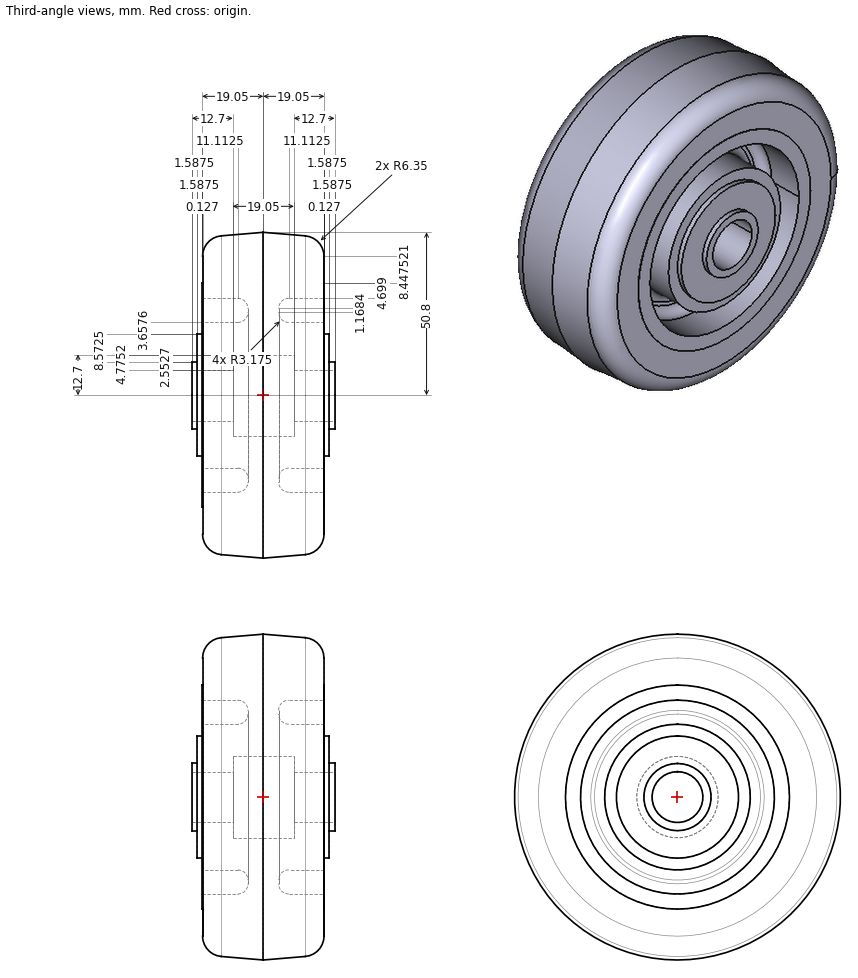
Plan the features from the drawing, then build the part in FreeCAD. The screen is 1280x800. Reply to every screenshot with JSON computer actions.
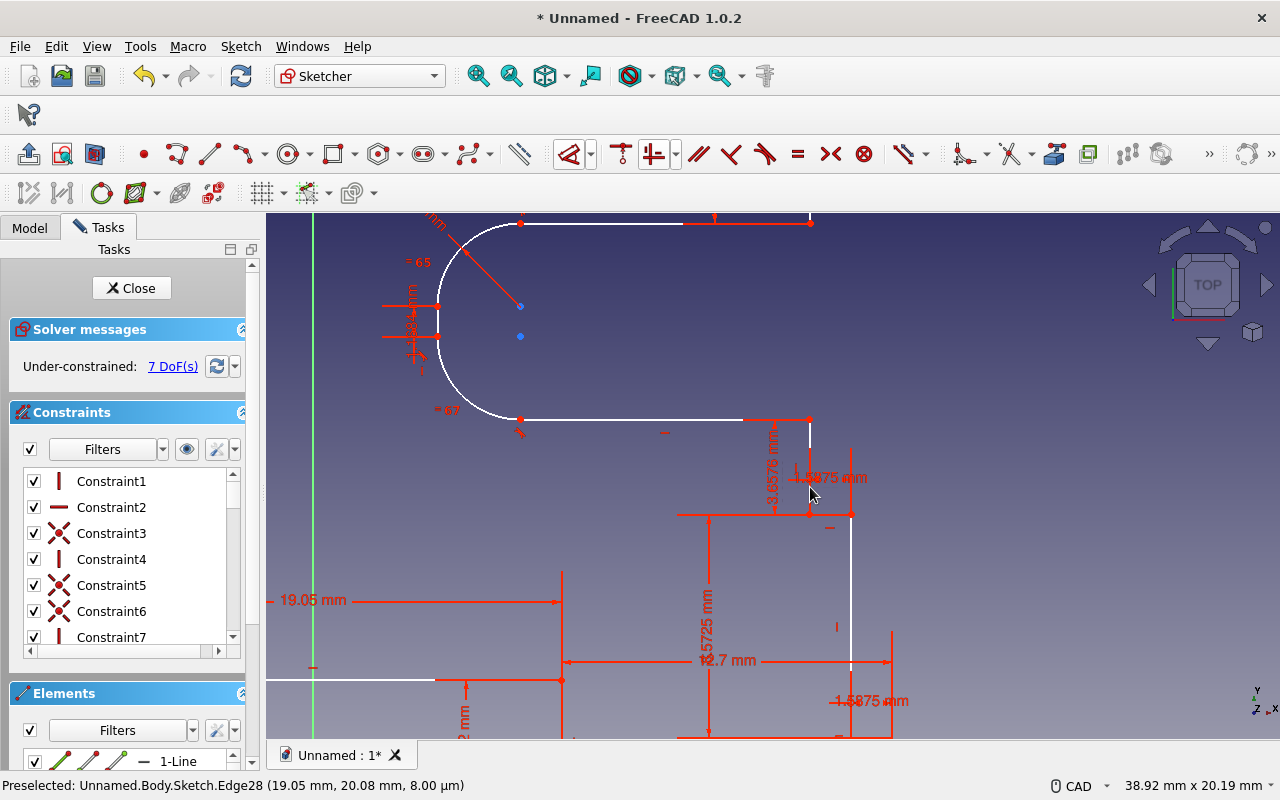
{"action": "scroll", "coordinate": [832, 517], "scroll_direction": "down", "scroll_amount": 7}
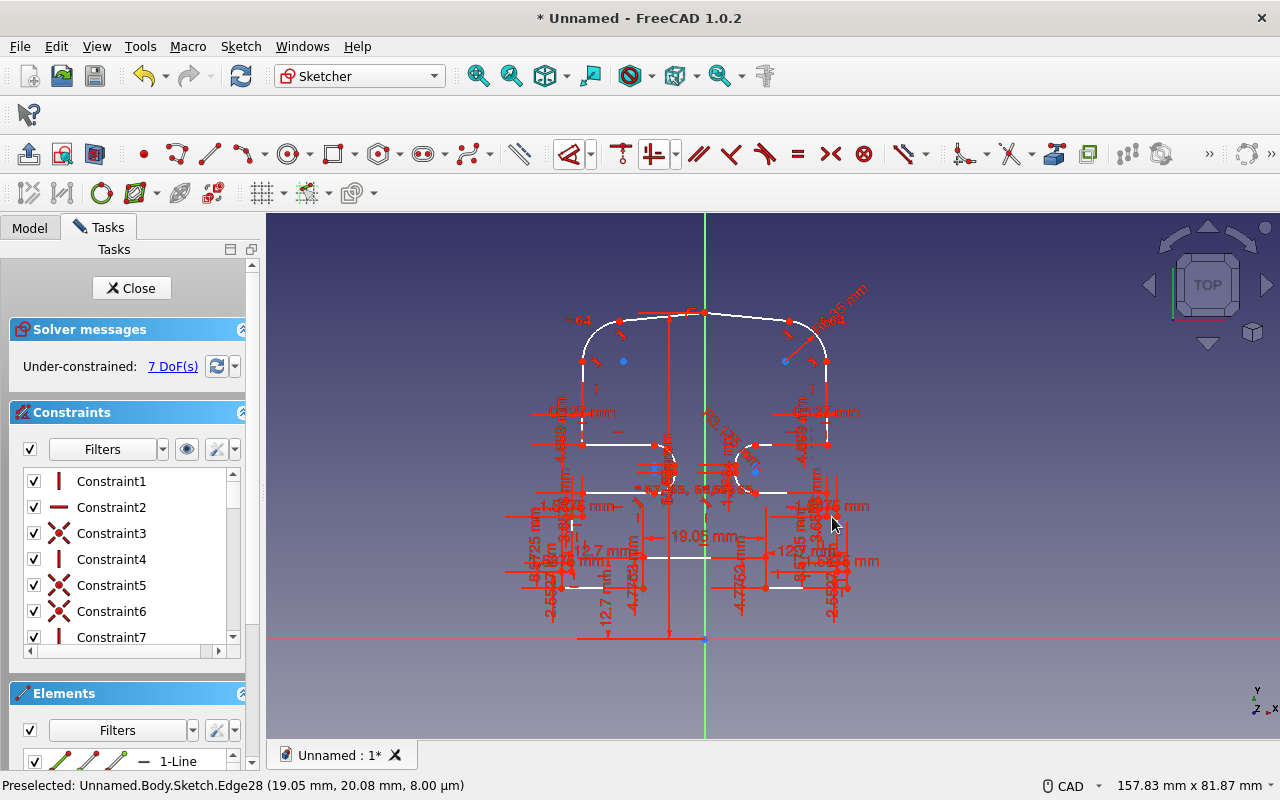
{"action": "left_click", "coordinate": [827, 445]}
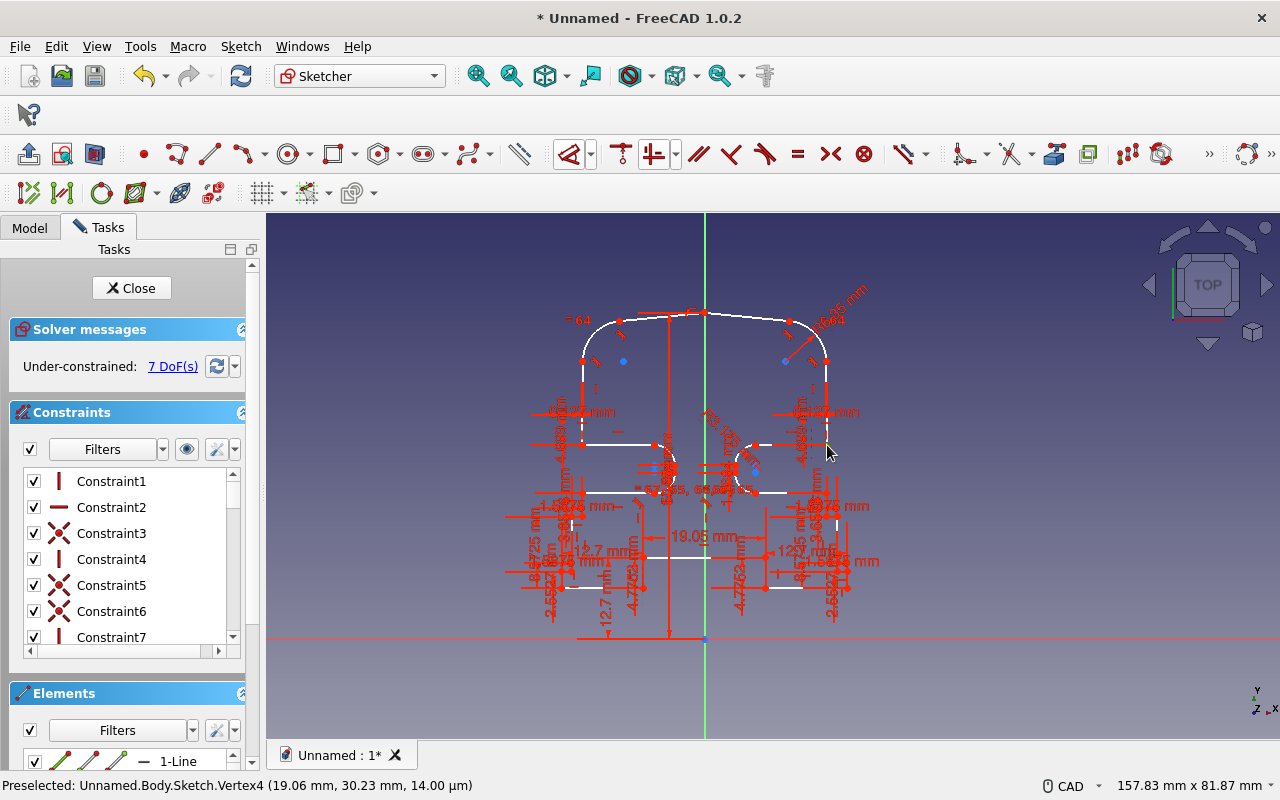
{"action": "left_click", "coordinate": [590, 154]}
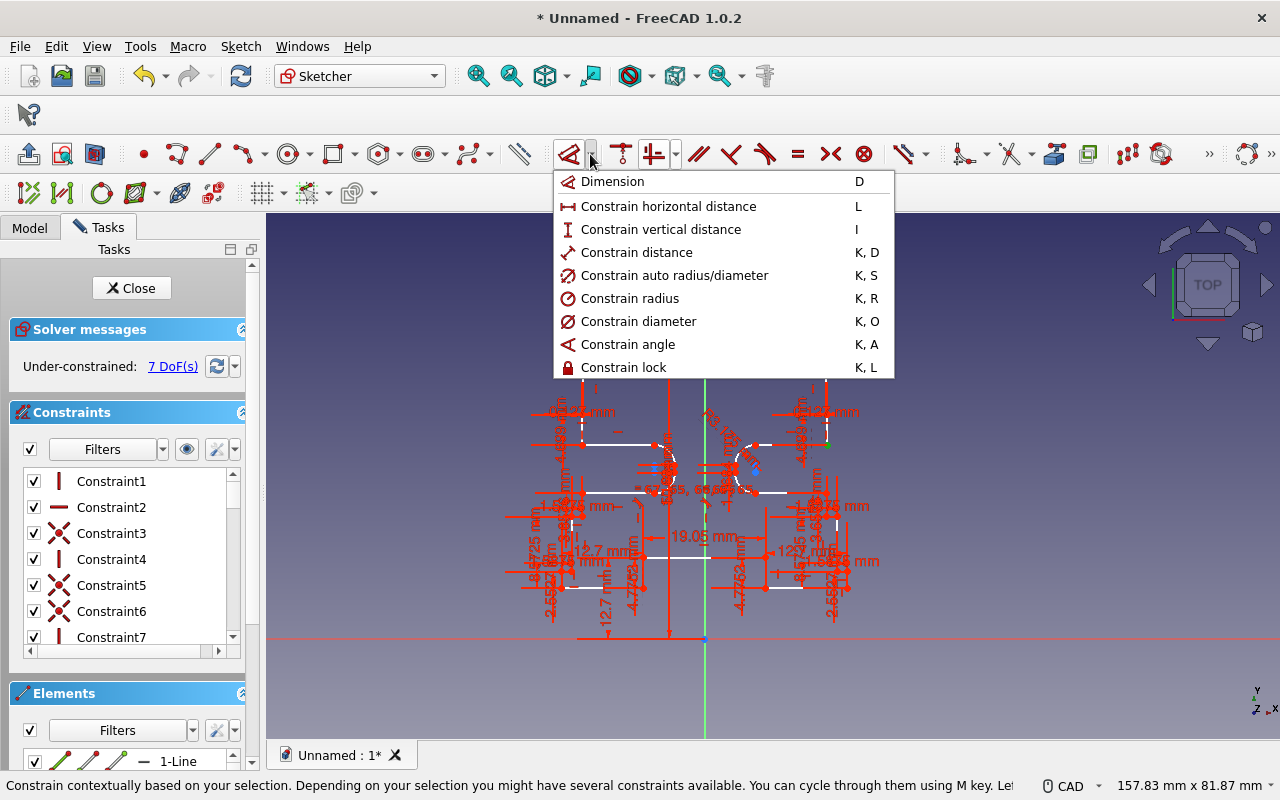
{"action": "left_click", "coordinate": [724, 206]}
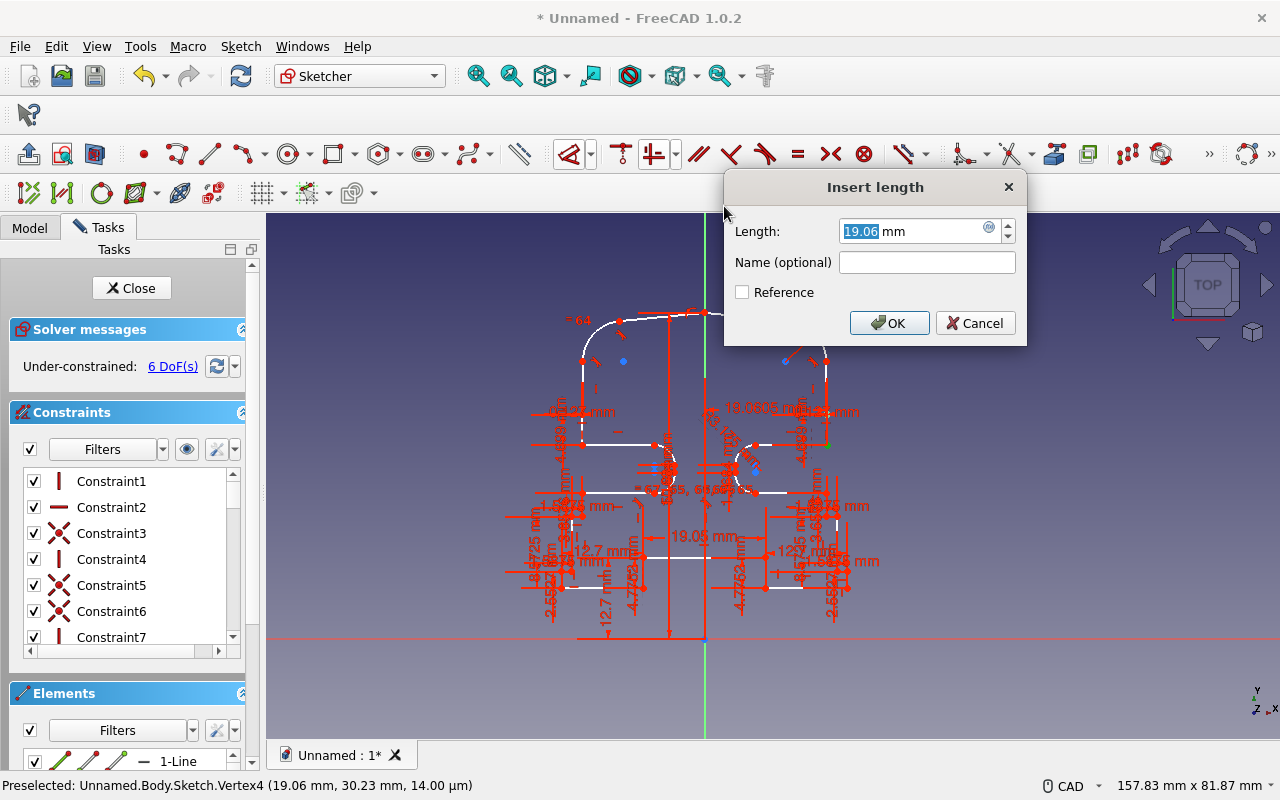
{"action": "type", "text": "19.05"}
{"action": "key", "text": "Return"}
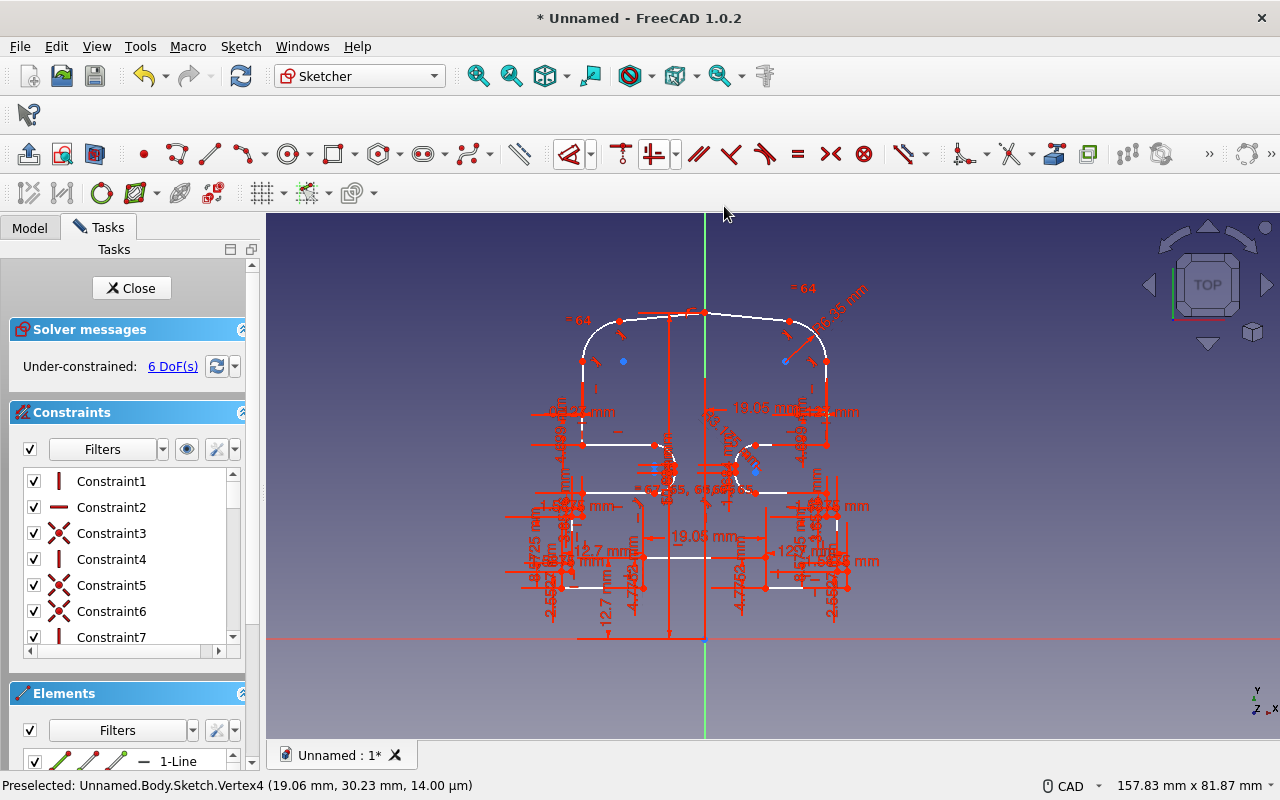
{"action": "scroll", "coordinate": [582, 415], "scroll_direction": "up", "scroll_amount": 14}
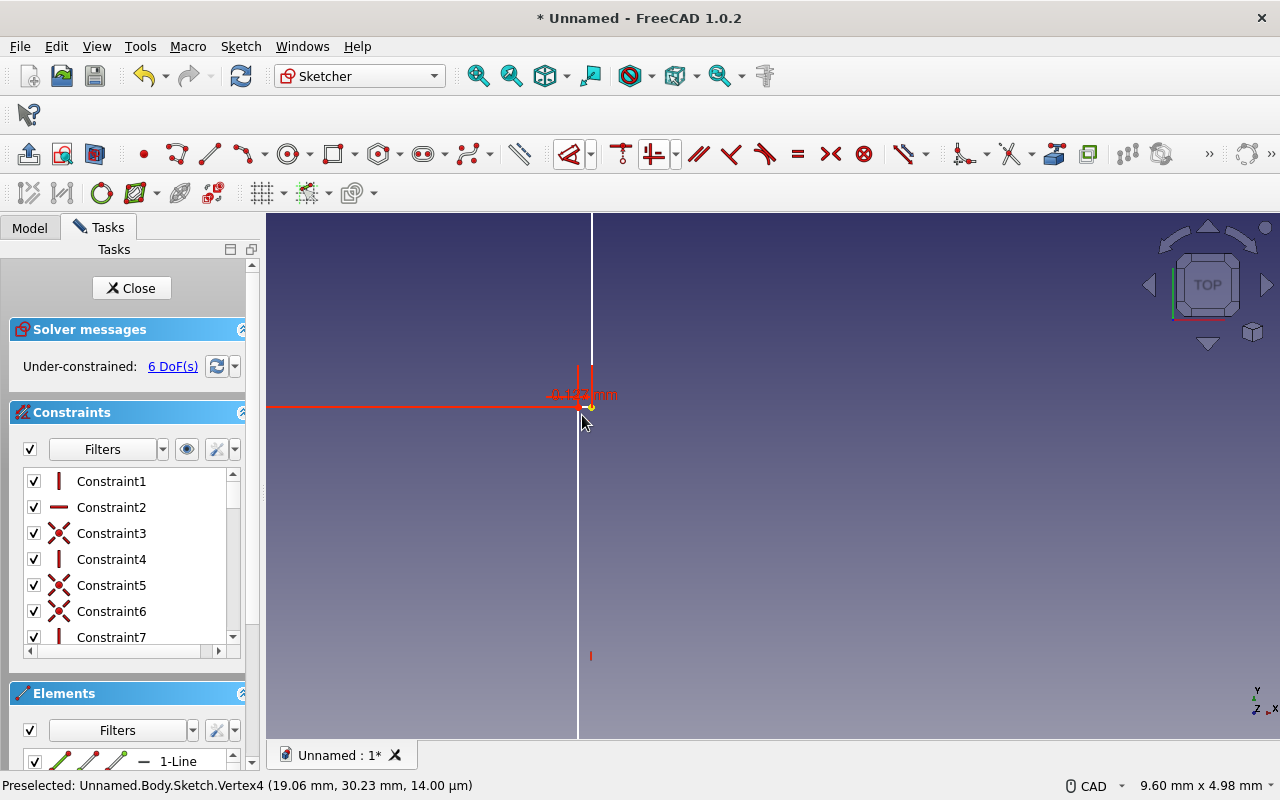
{"action": "left_click", "coordinate": [578, 407]}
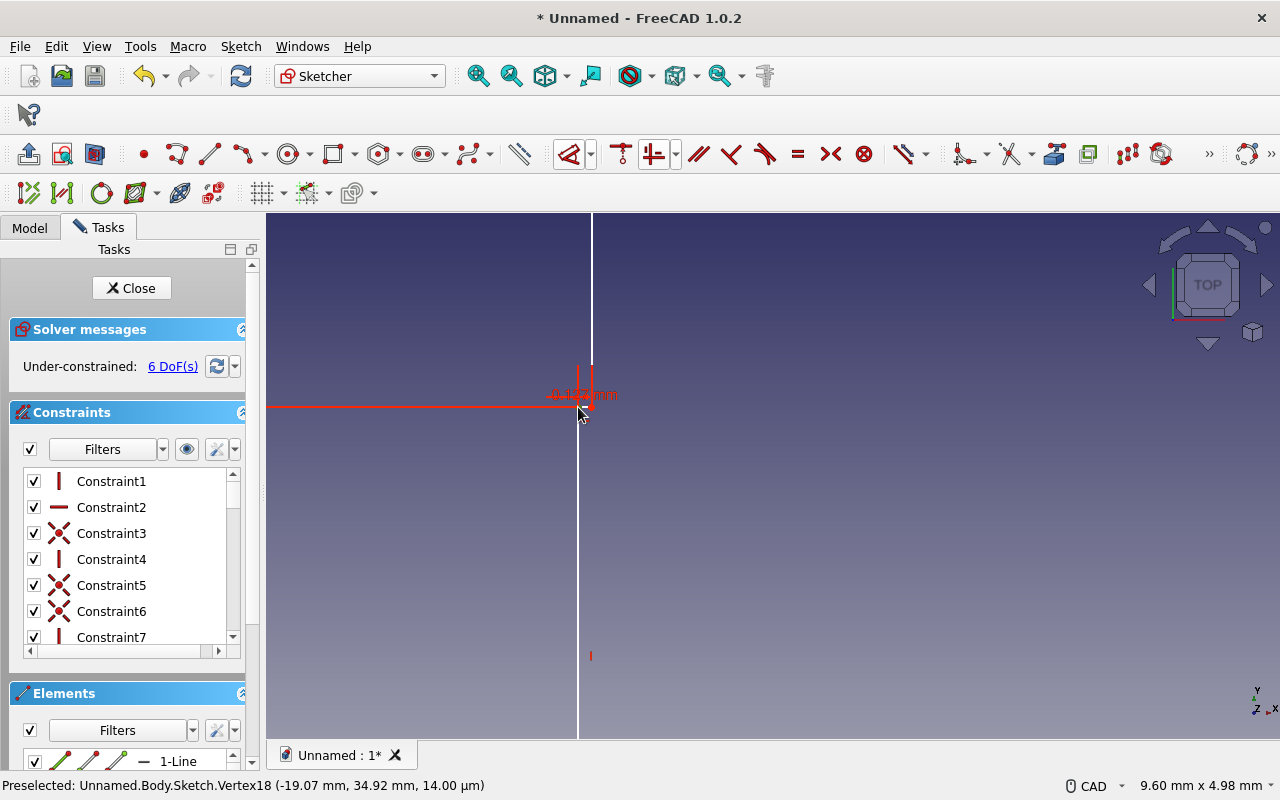
{"action": "left_click", "coordinate": [590, 154]}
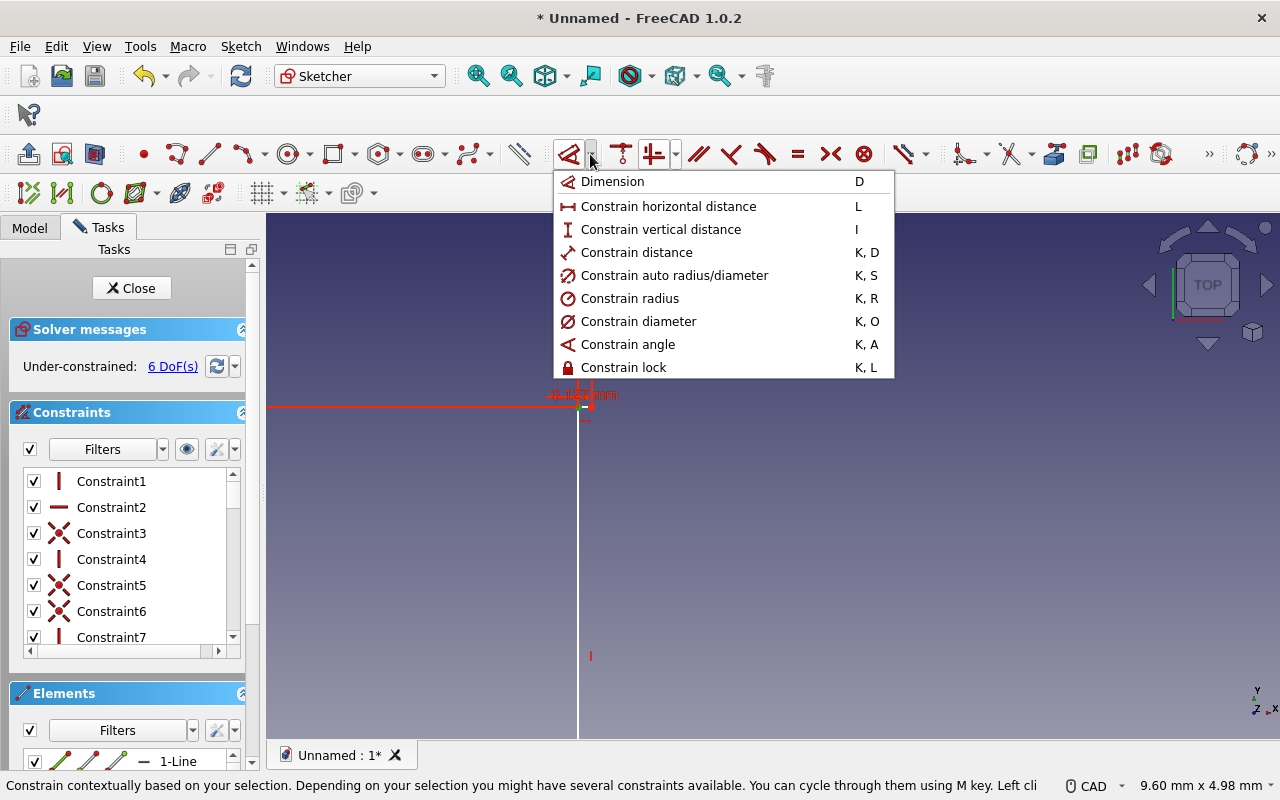
{"action": "left_click", "coordinate": [724, 206]}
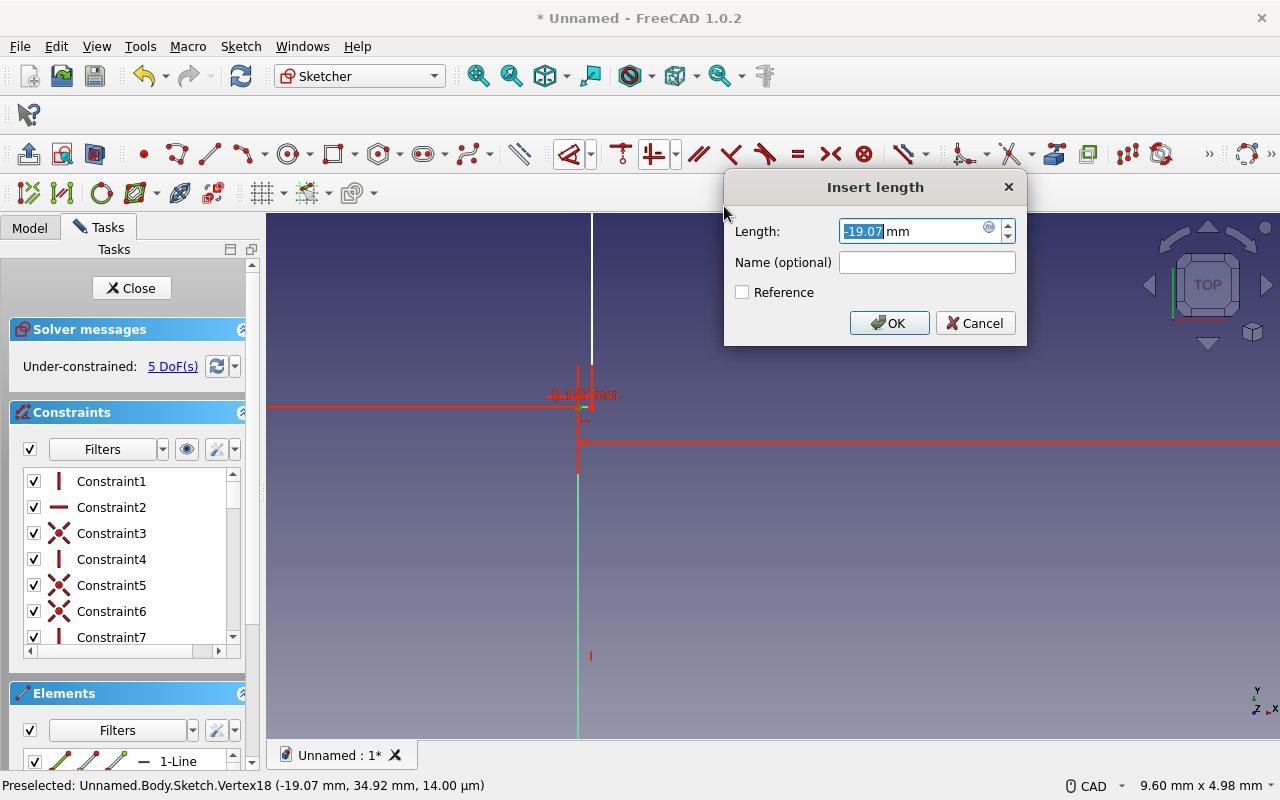
{"action": "type", "text": "-19.05"}
{"action": "key", "text": "Return"}